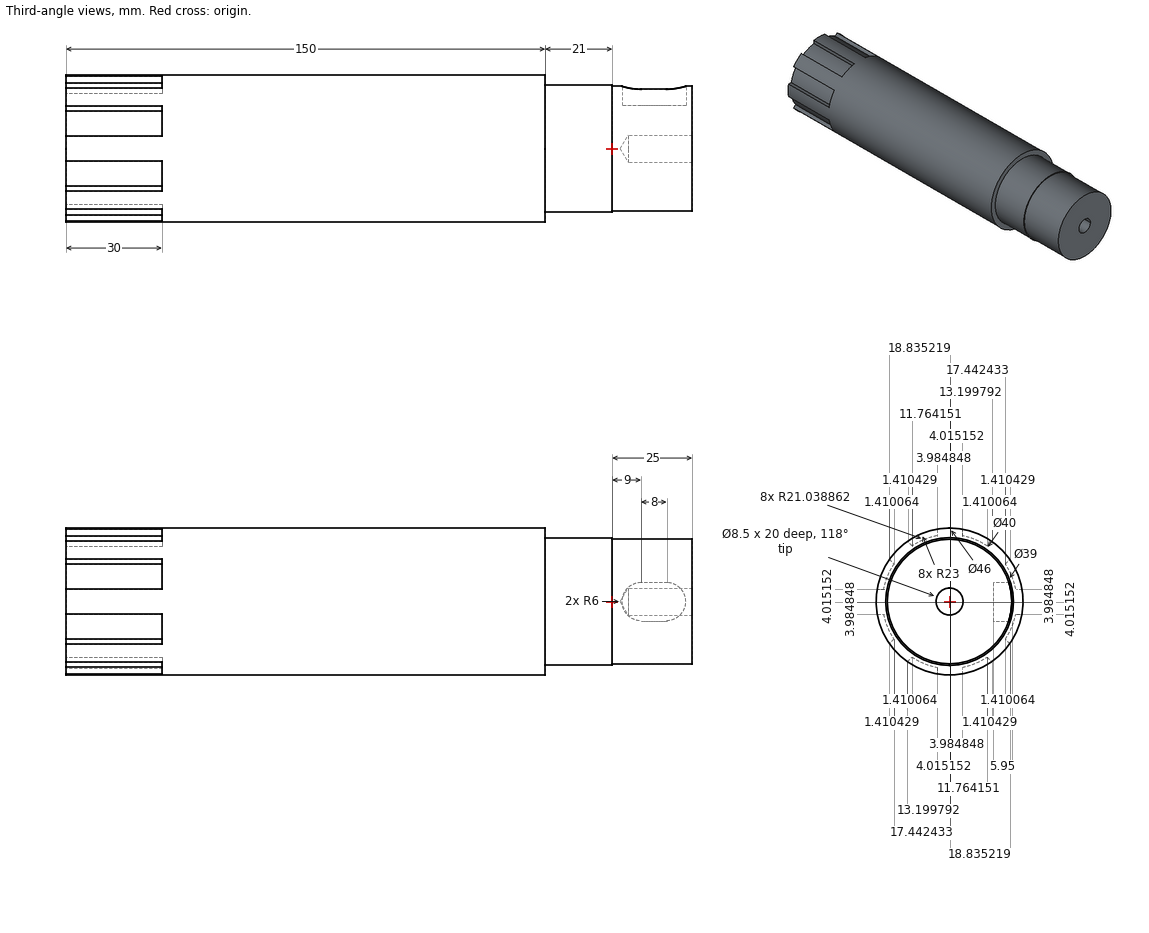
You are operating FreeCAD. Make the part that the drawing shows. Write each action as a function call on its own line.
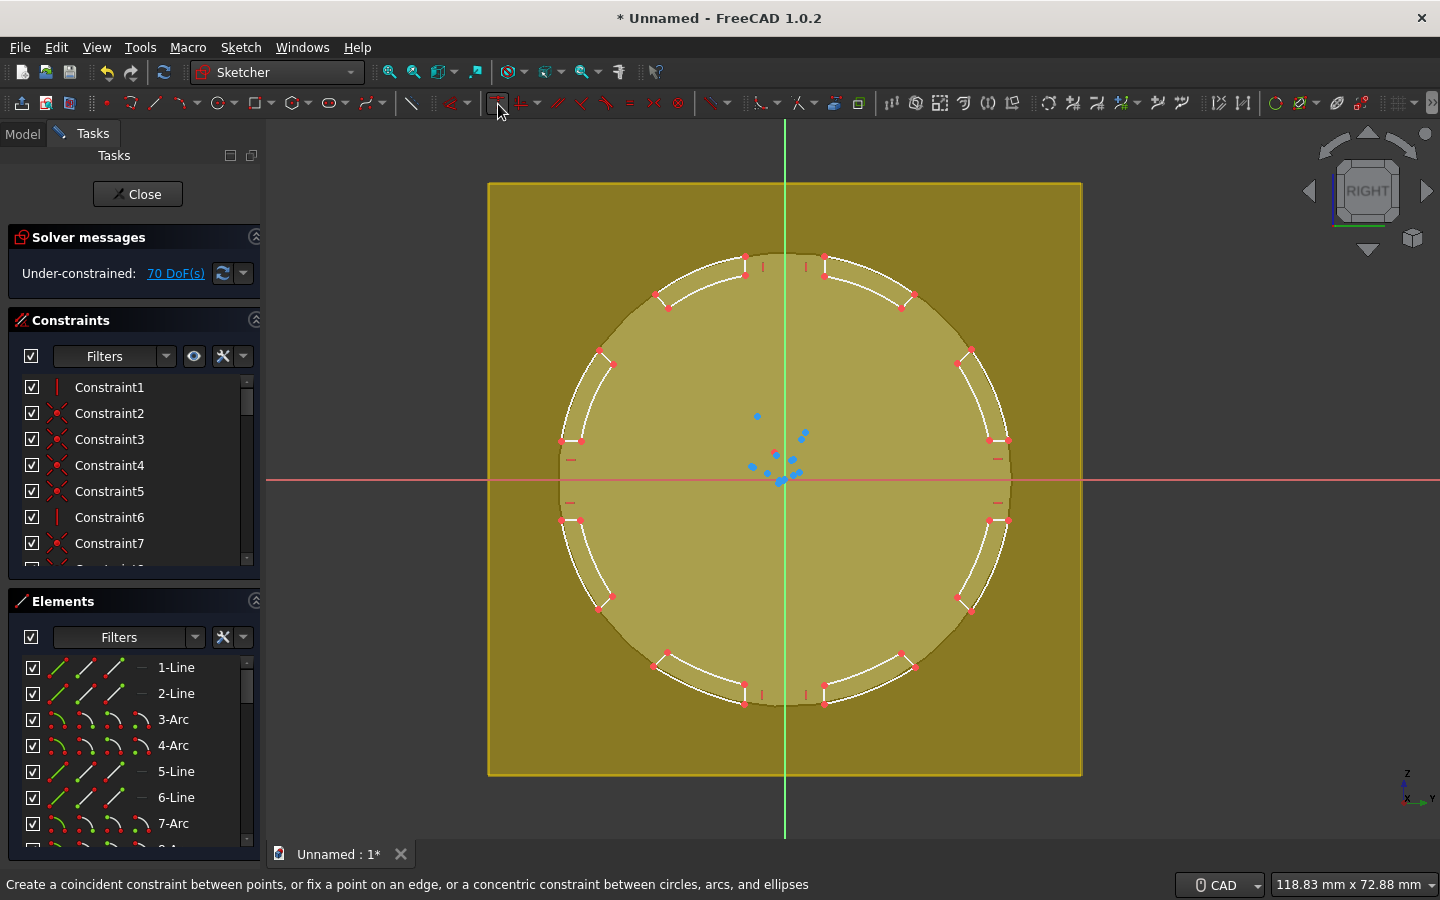
click(721, 282)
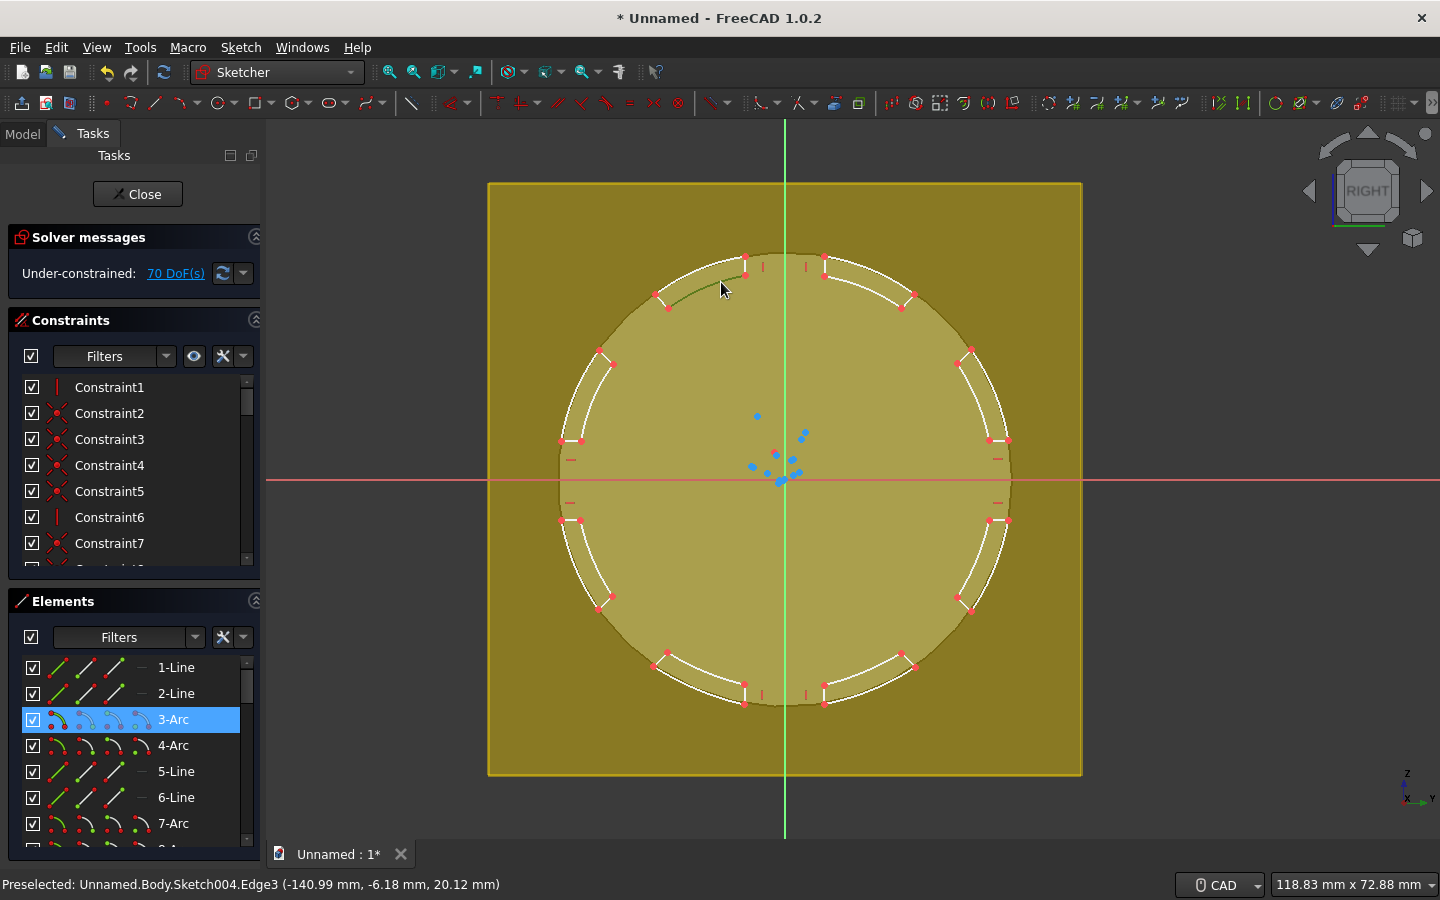
click(880, 295)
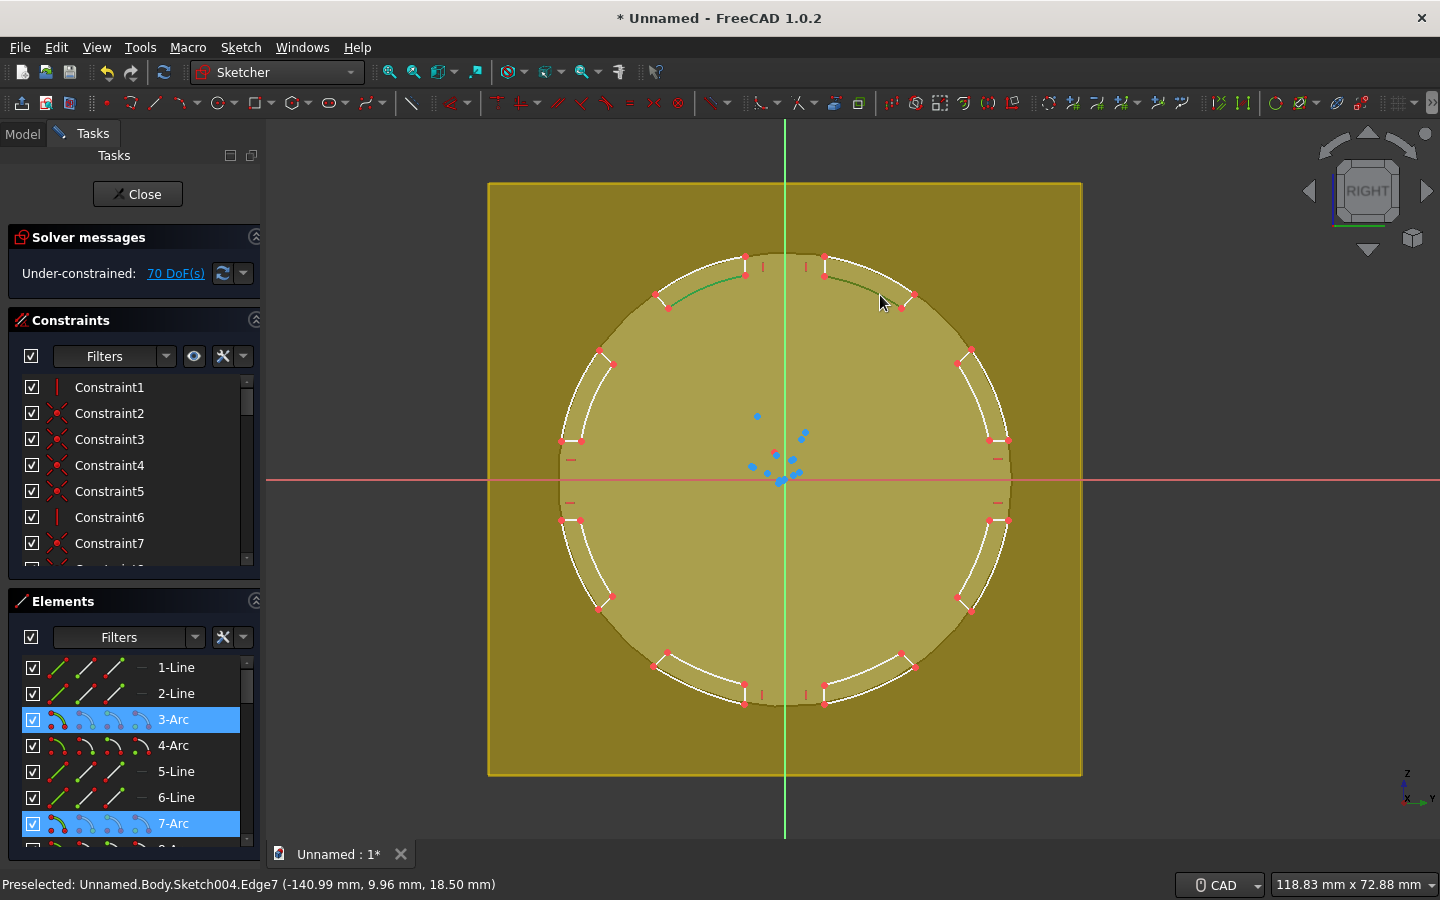
click(498, 104)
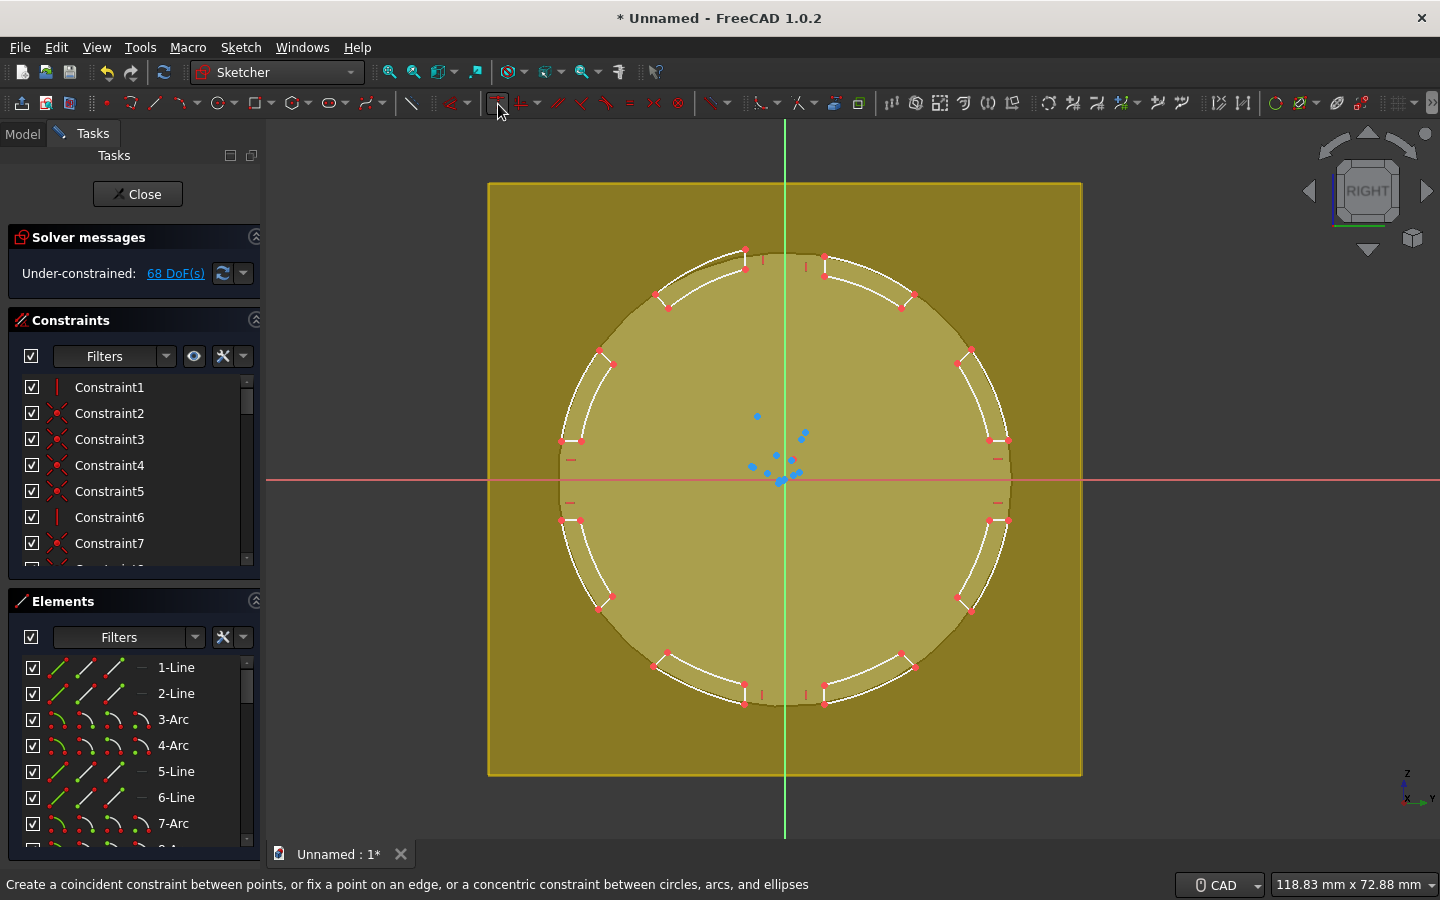
click(720, 278)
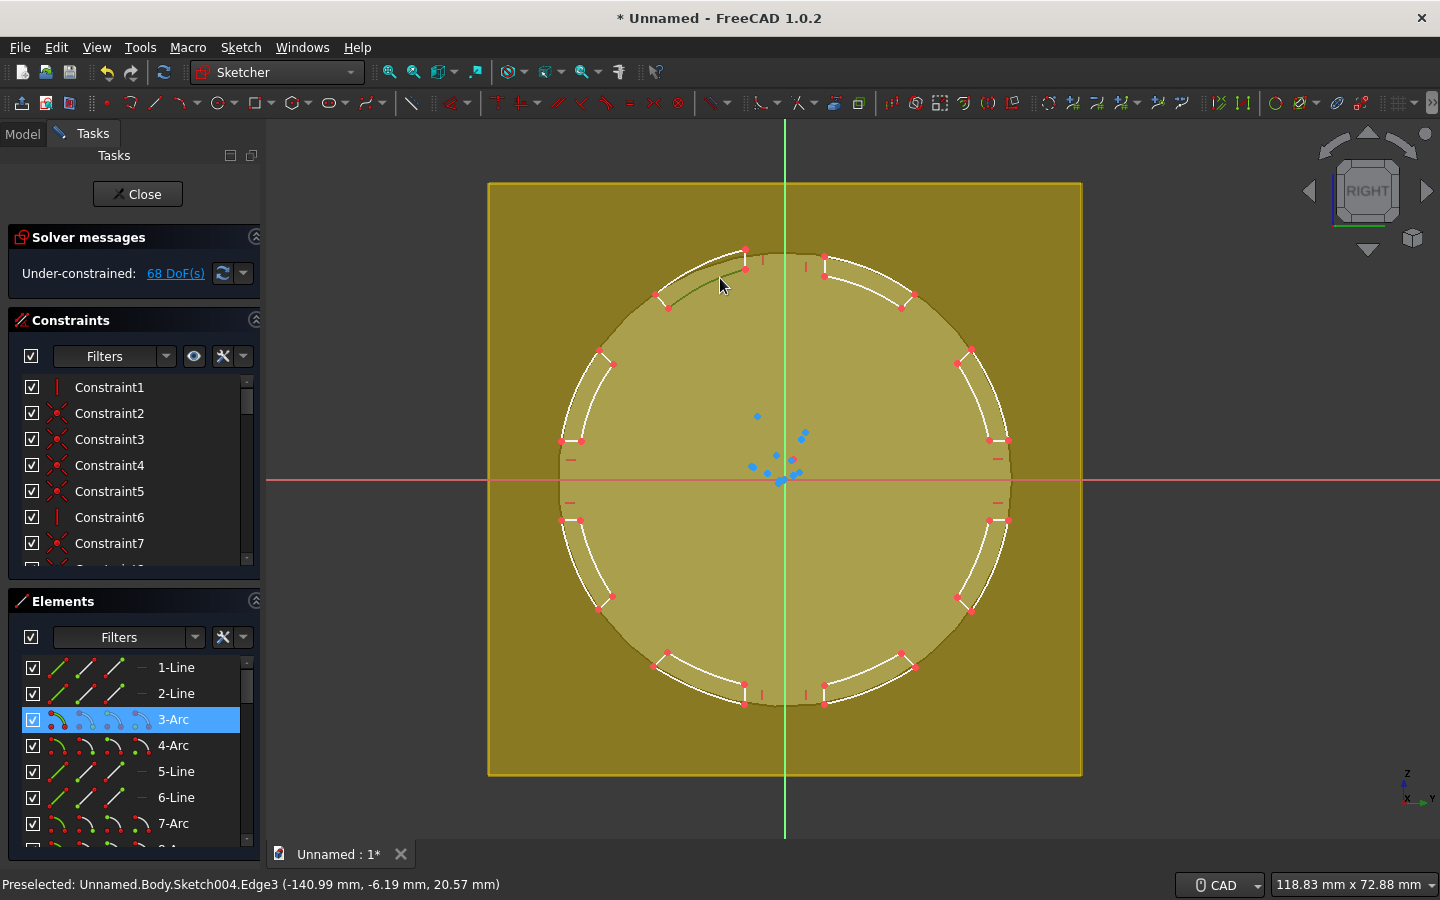
click(890, 279)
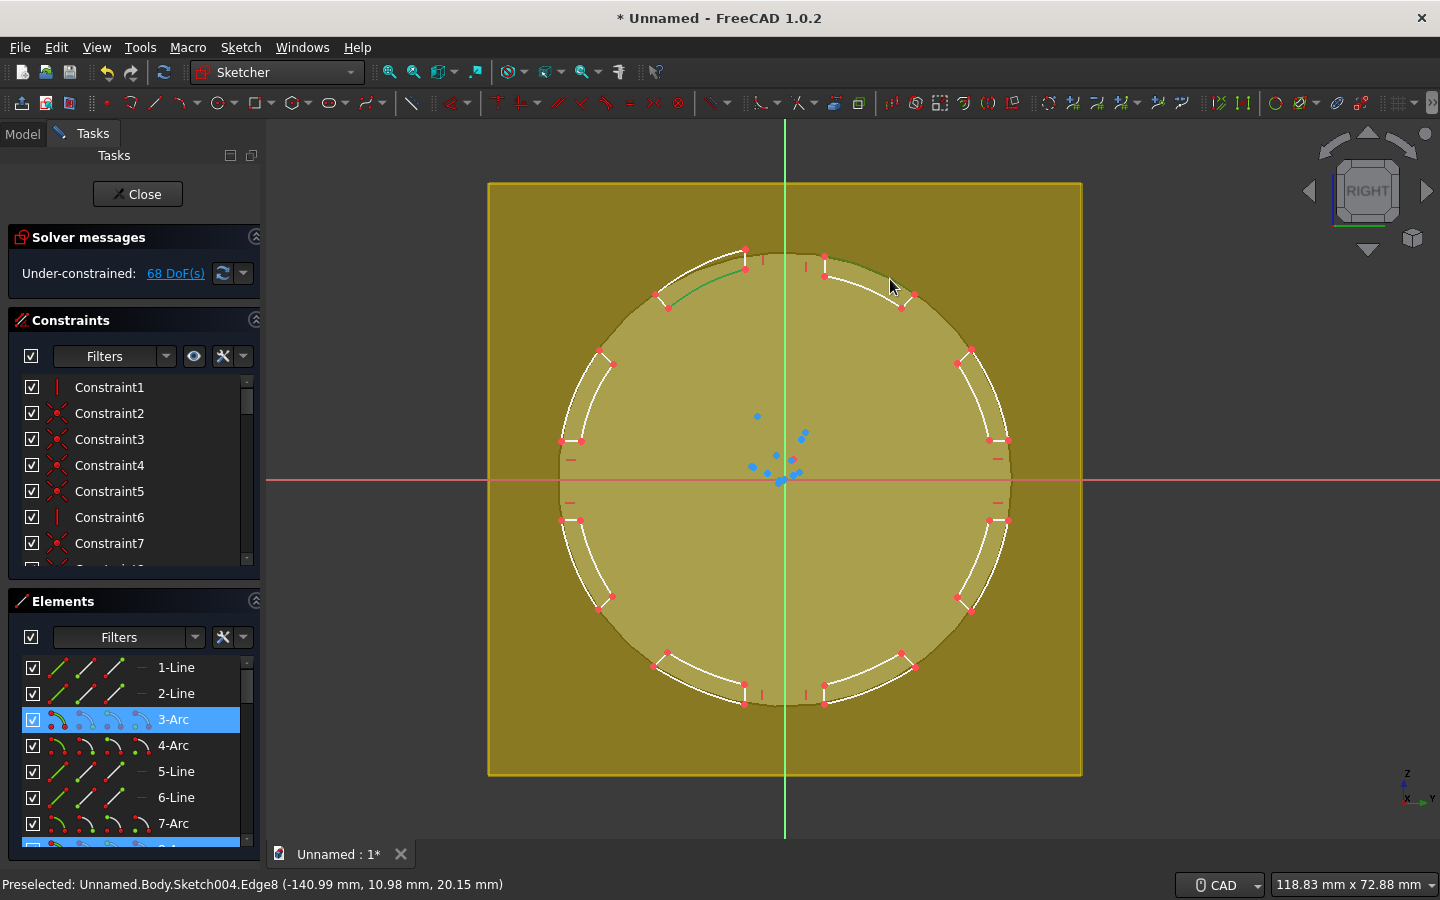
click(498, 104)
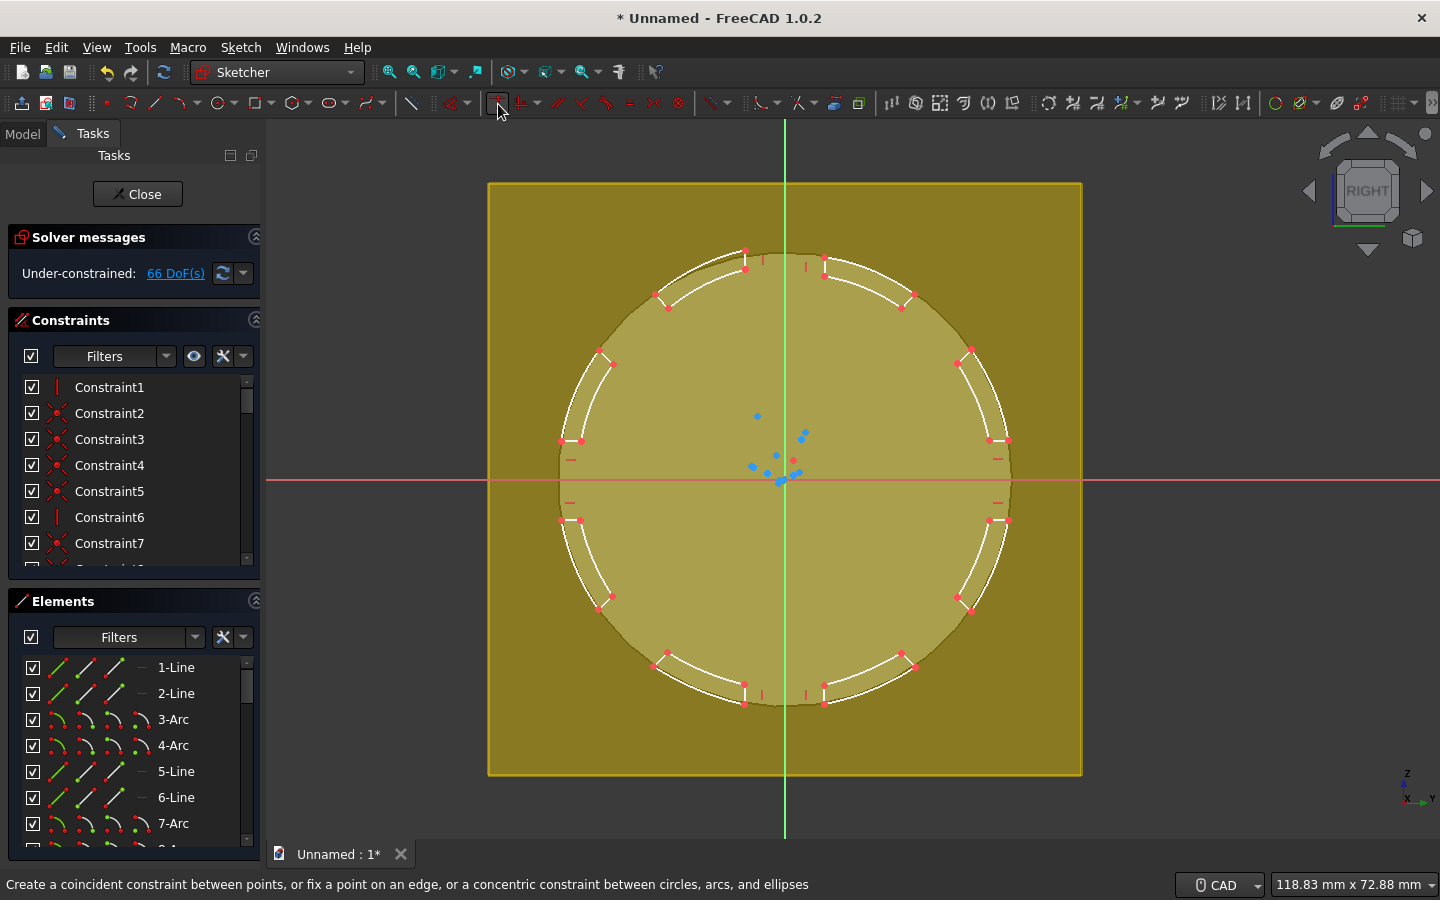
click(720, 278)